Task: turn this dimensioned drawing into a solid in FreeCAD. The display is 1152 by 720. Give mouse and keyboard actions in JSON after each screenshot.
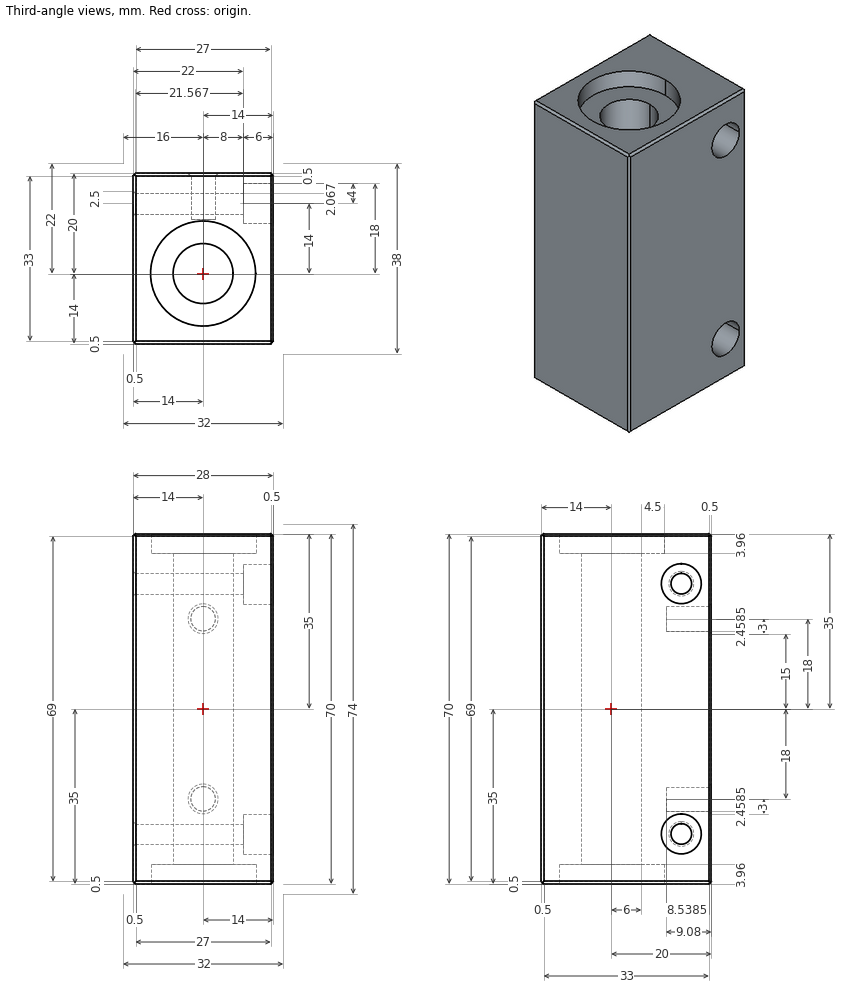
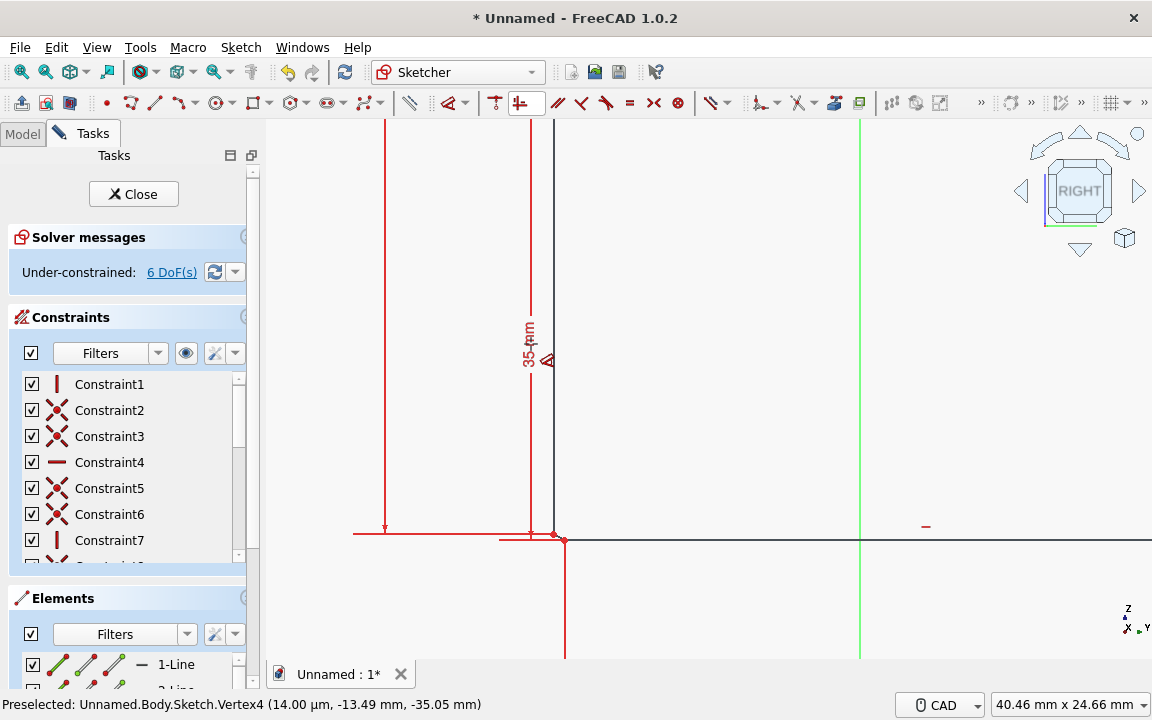
{"action": "scroll", "coordinate": [568, 545], "scroll_direction": "down", "scroll_amount": 8}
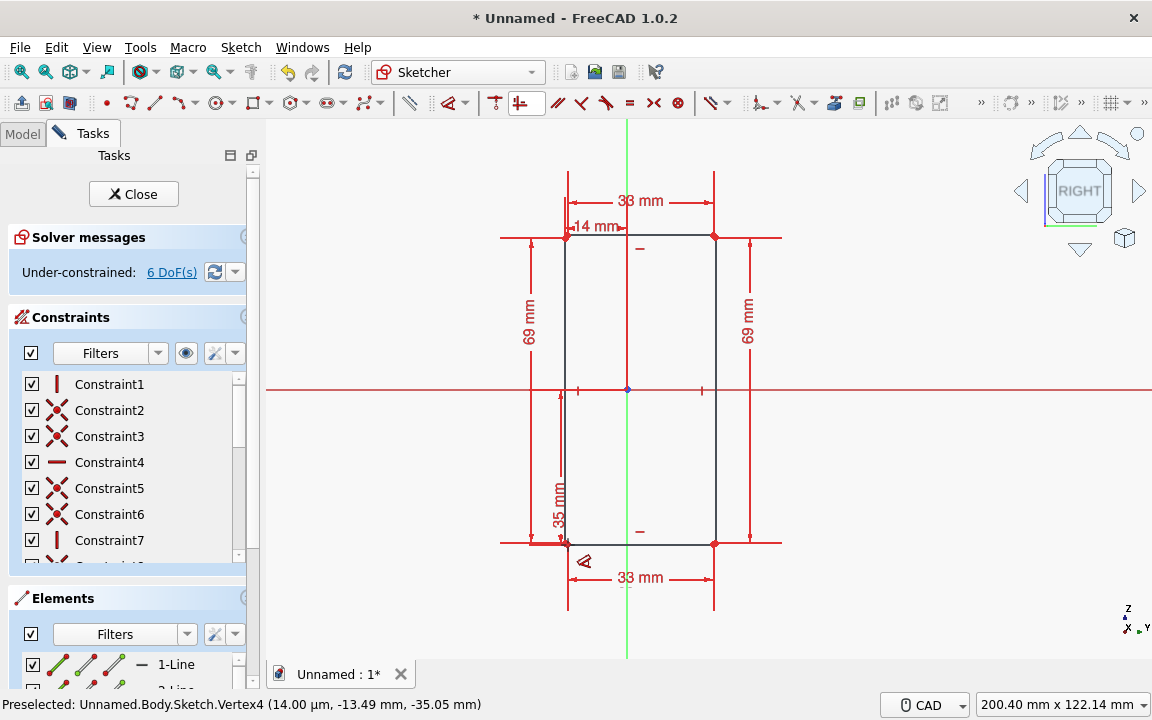
{"action": "scroll", "coordinate": [716, 543], "scroll_direction": "up", "scroll_amount": 8}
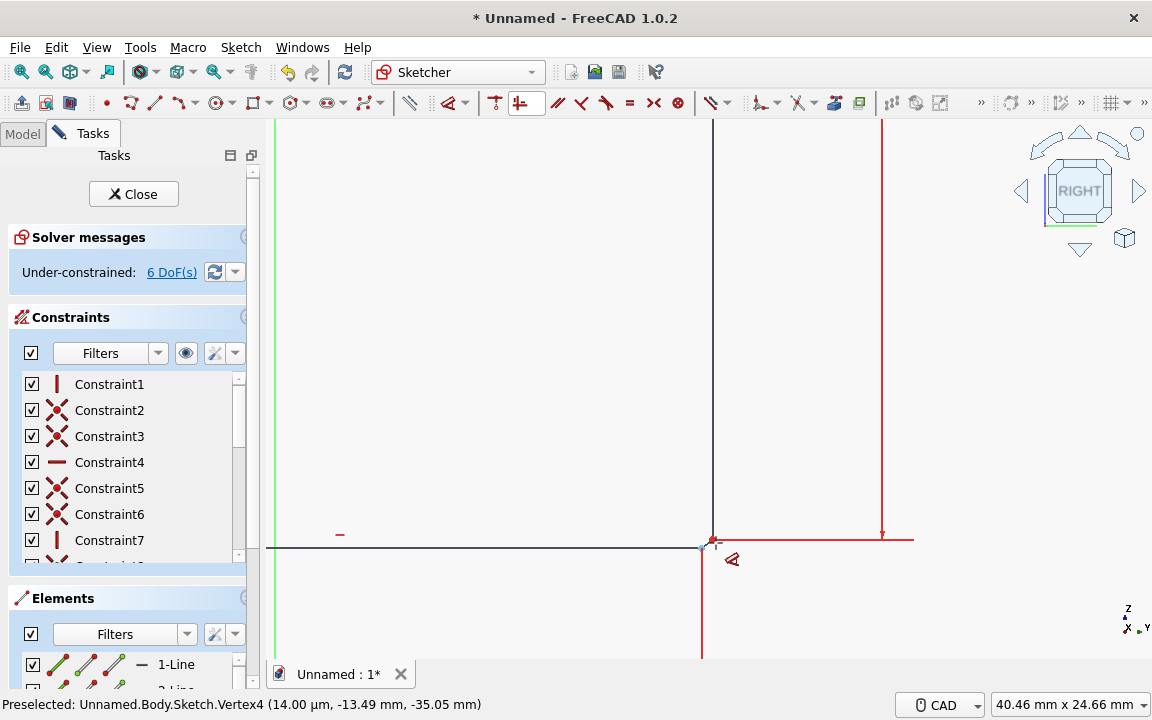
{"action": "left_click", "coordinate": [713, 540]}
{"action": "left_click", "coordinate": [503, 574]}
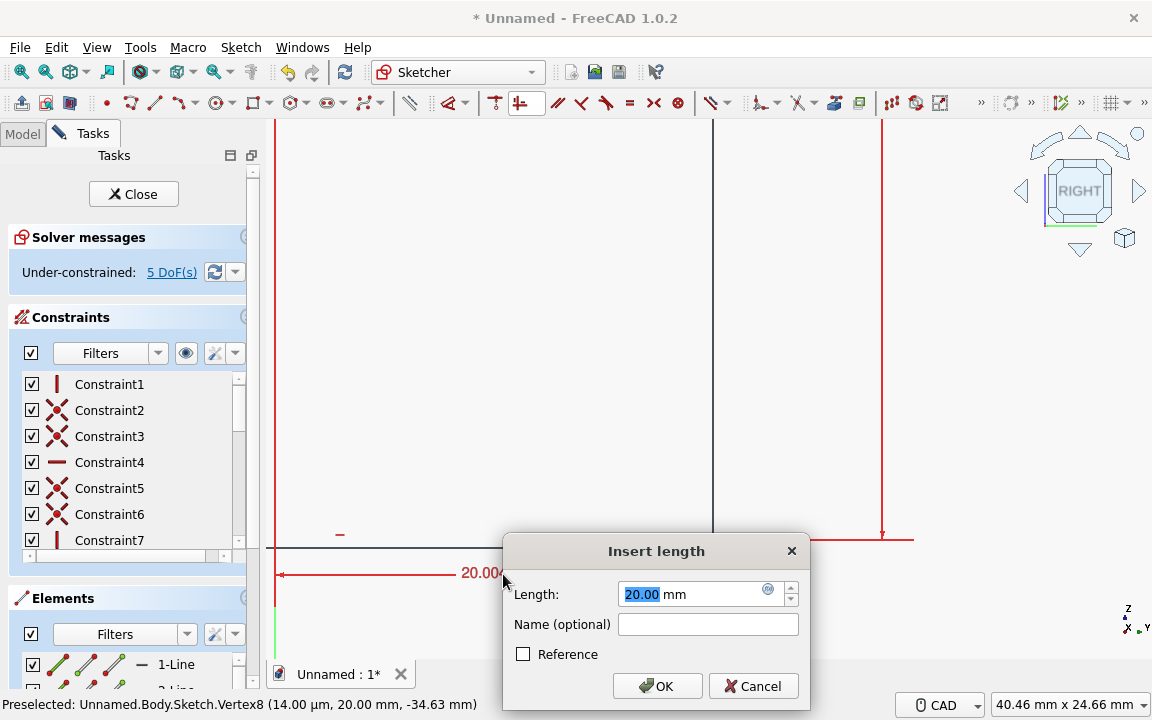
{"action": "type", "text": "20"}
{"action": "key", "text": "Return"}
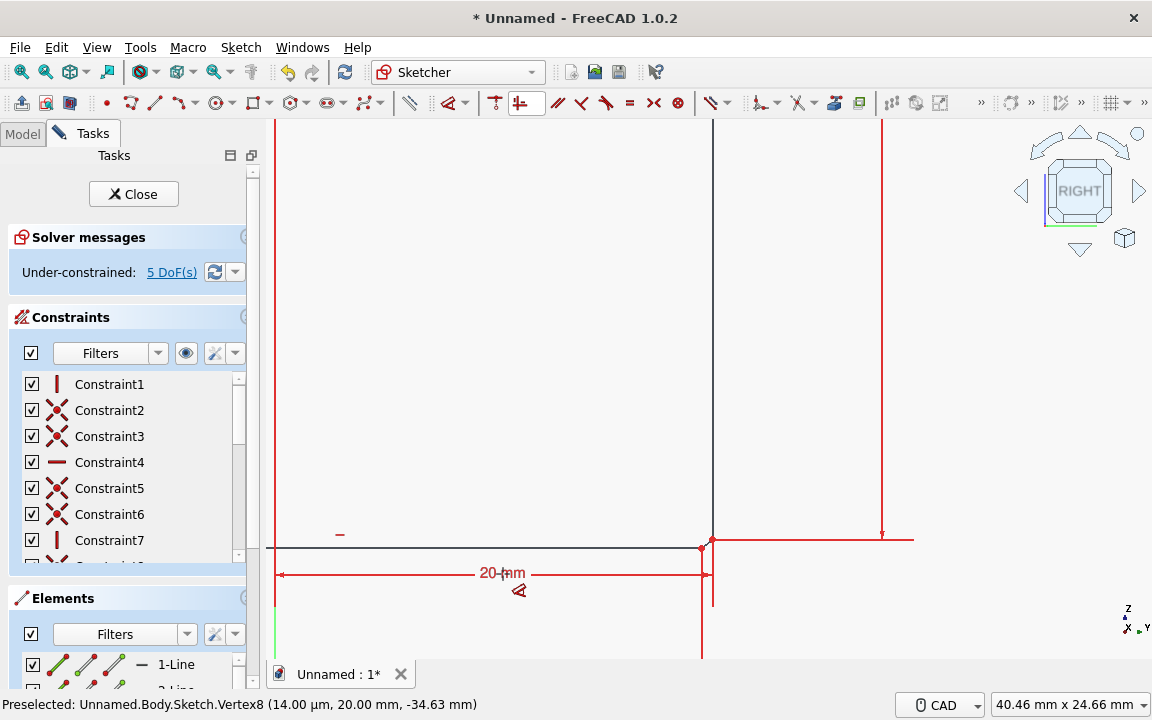
{"action": "scroll", "coordinate": [716, 543], "scroll_direction": "down", "scroll_amount": 8}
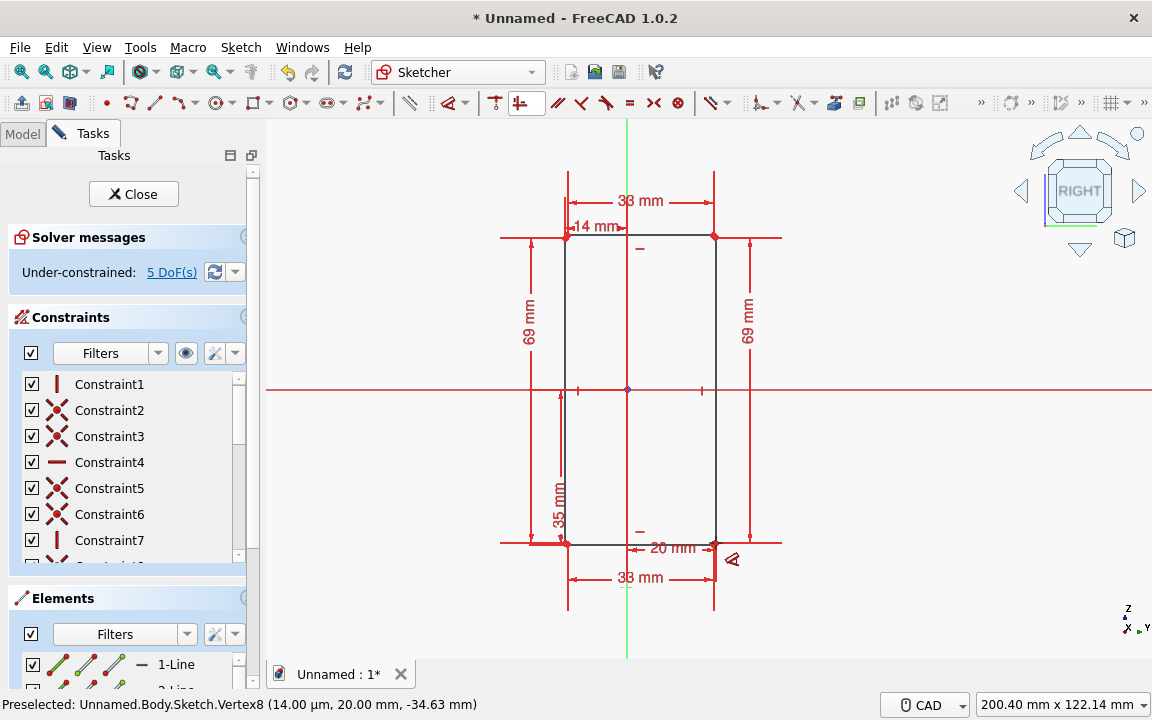
{"action": "scroll", "coordinate": [714, 235], "scroll_direction": "up", "scroll_amount": 7}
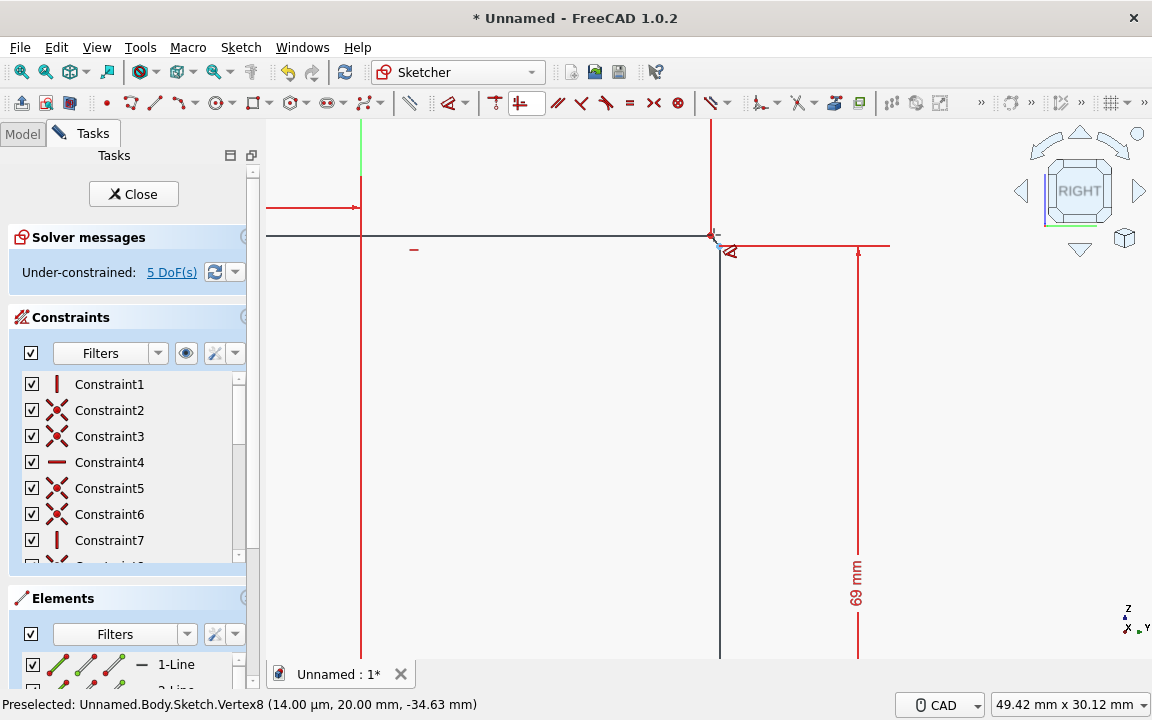
{"action": "left_click", "coordinate": [711, 236]}
{"action": "left_click", "coordinate": [745, 433]}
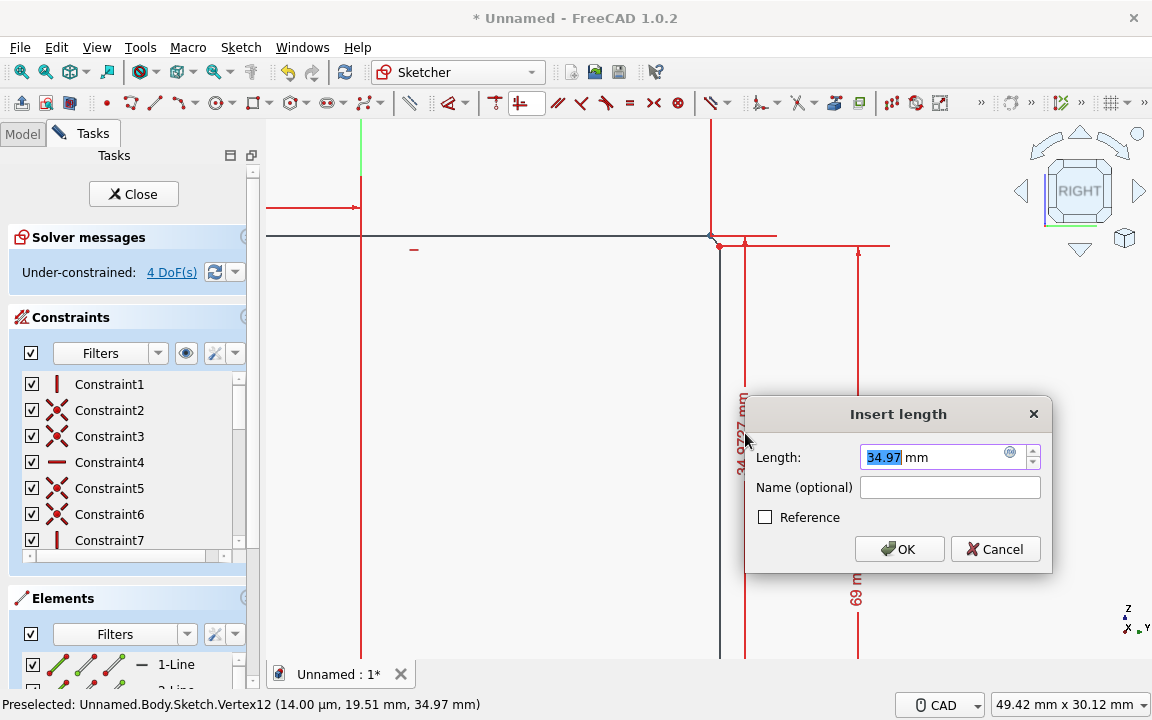
{"action": "type", "text": "35"}
{"action": "key", "text": "Return"}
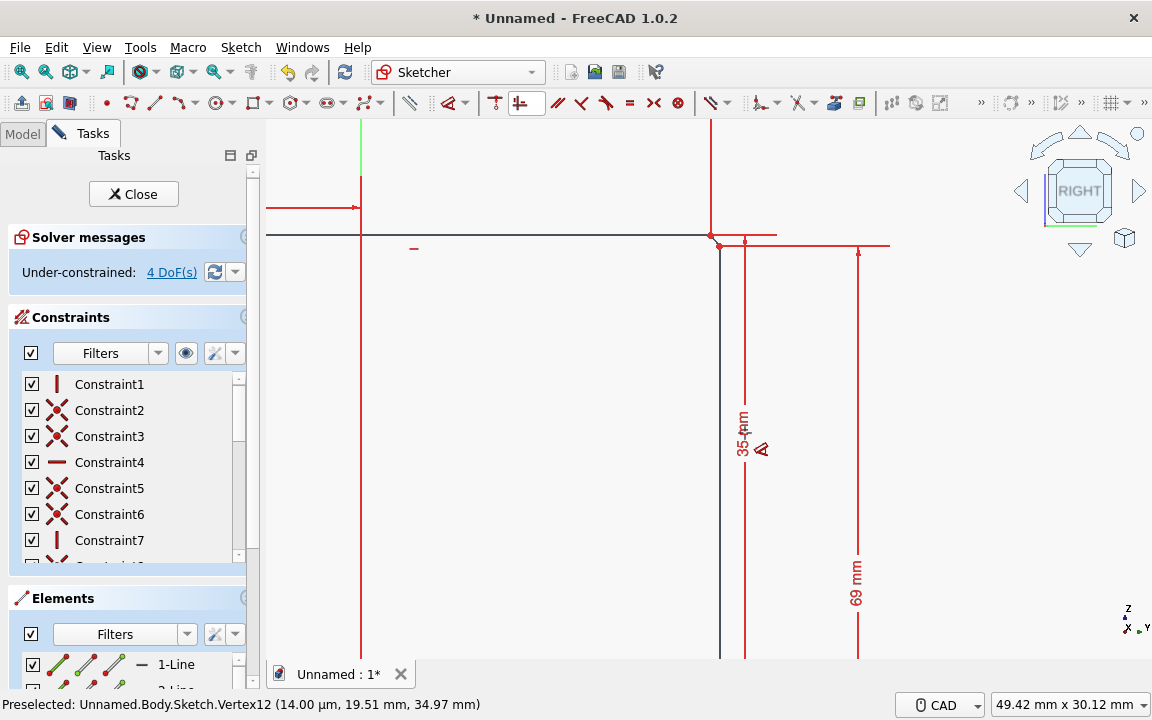
{"action": "scroll", "coordinate": [714, 234], "scroll_direction": "down", "scroll_amount": 7}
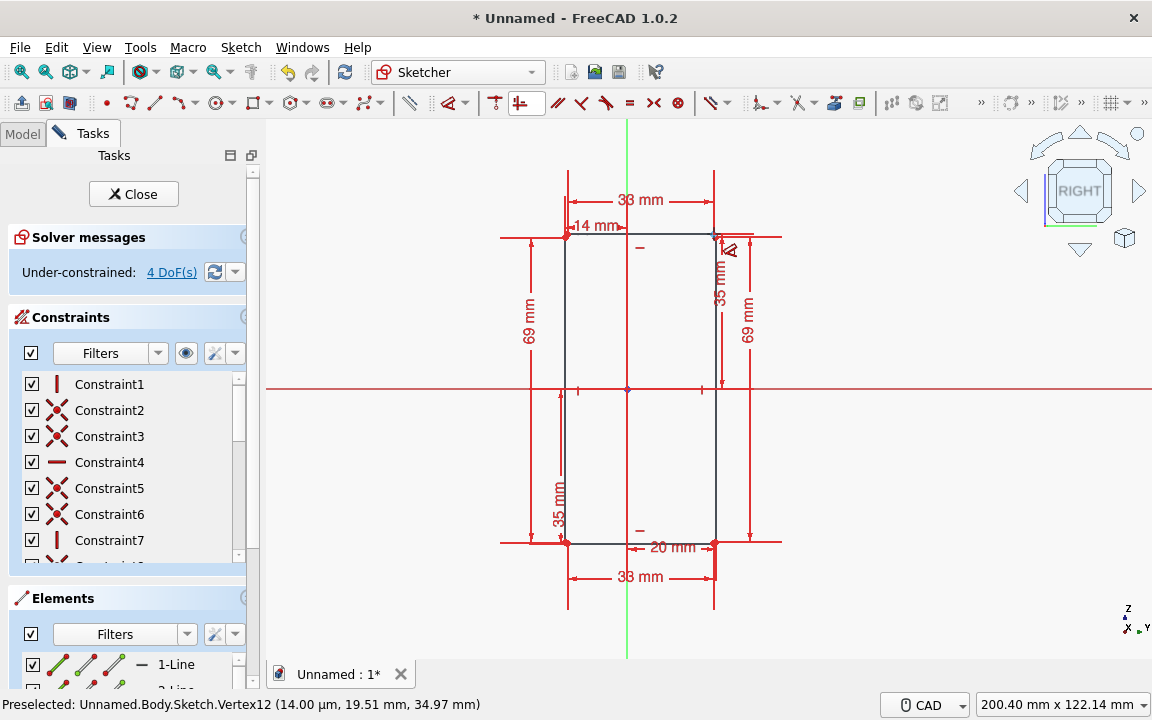
{"action": "scroll", "coordinate": [567, 543], "scroll_direction": "up", "scroll_amount": 15}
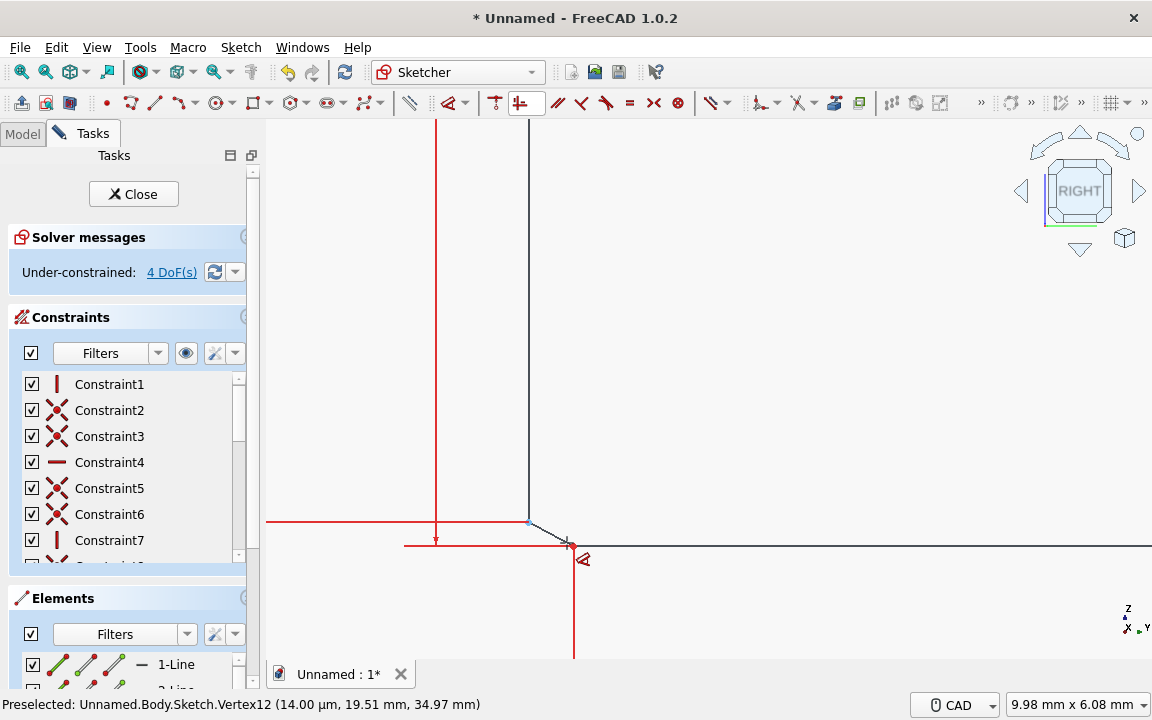
{"action": "left_click", "coordinate": [551, 534]}
{"action": "left_click", "coordinate": [551, 580]}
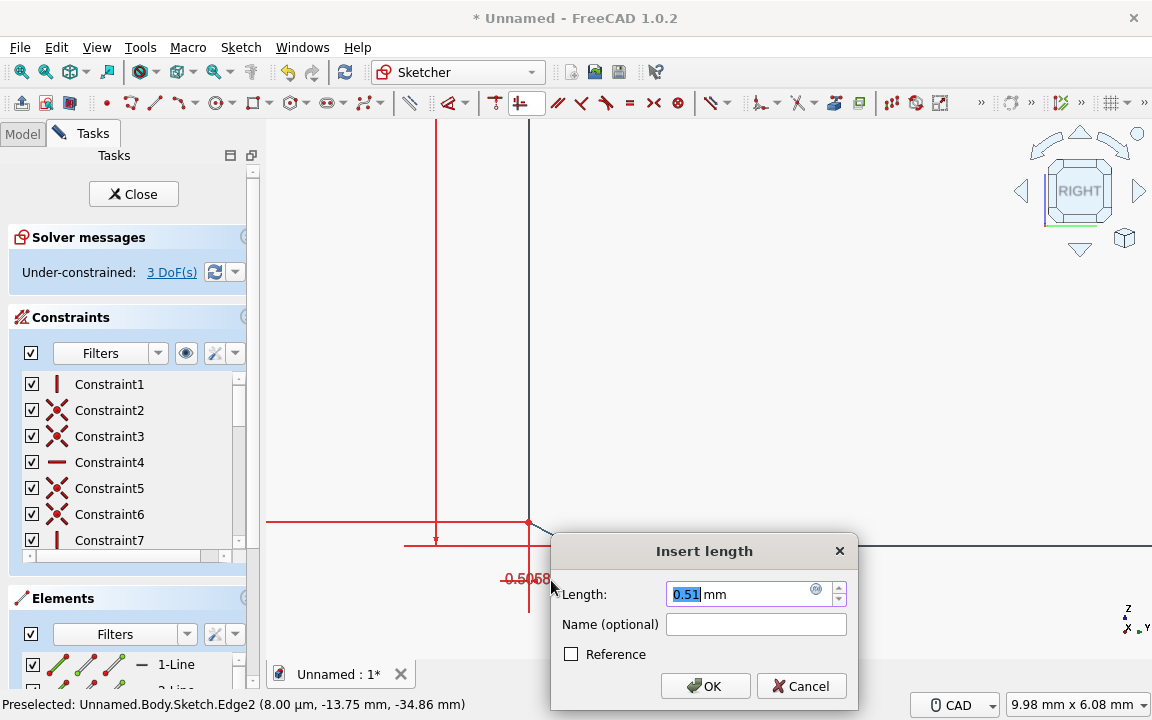
{"action": "type", "text": "0.5"}
{"action": "key", "text": "Return"}